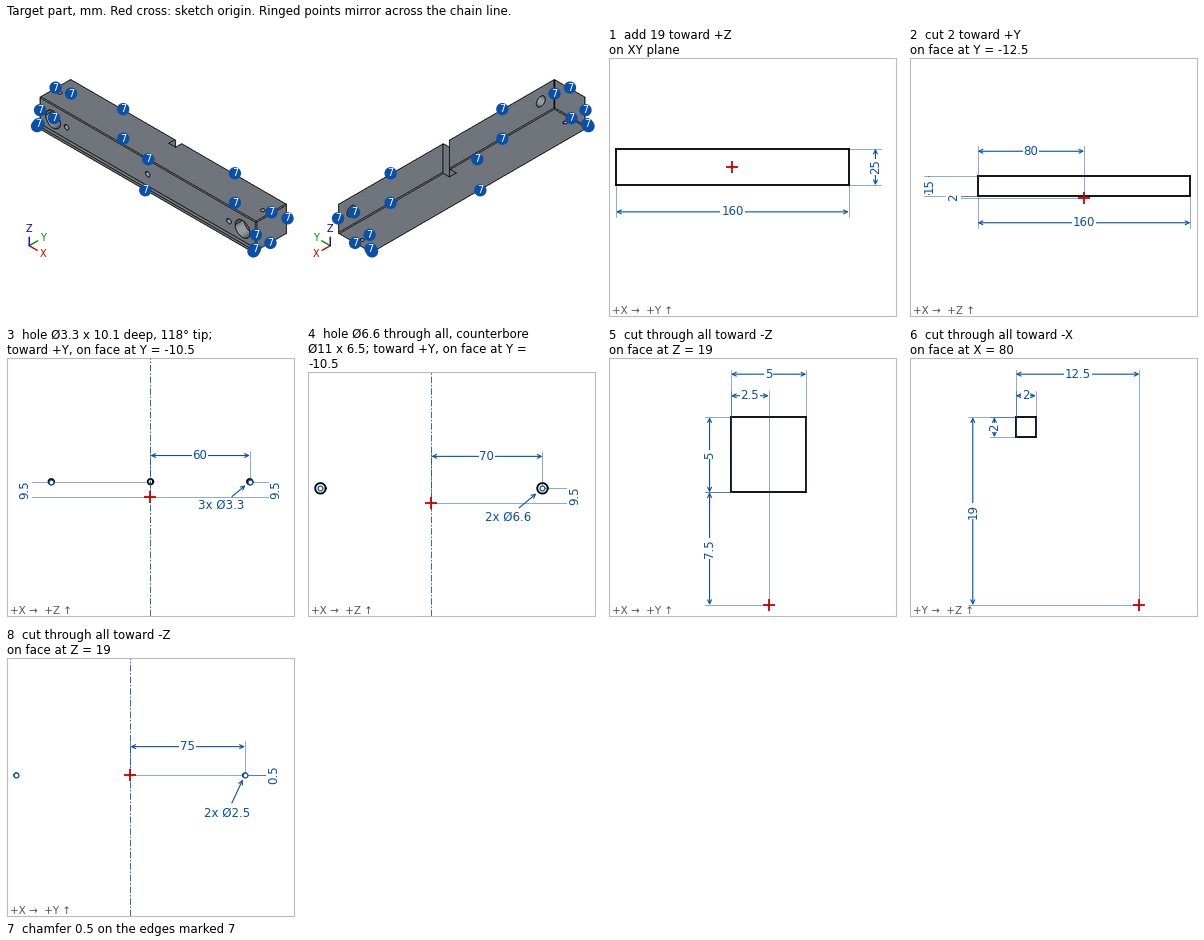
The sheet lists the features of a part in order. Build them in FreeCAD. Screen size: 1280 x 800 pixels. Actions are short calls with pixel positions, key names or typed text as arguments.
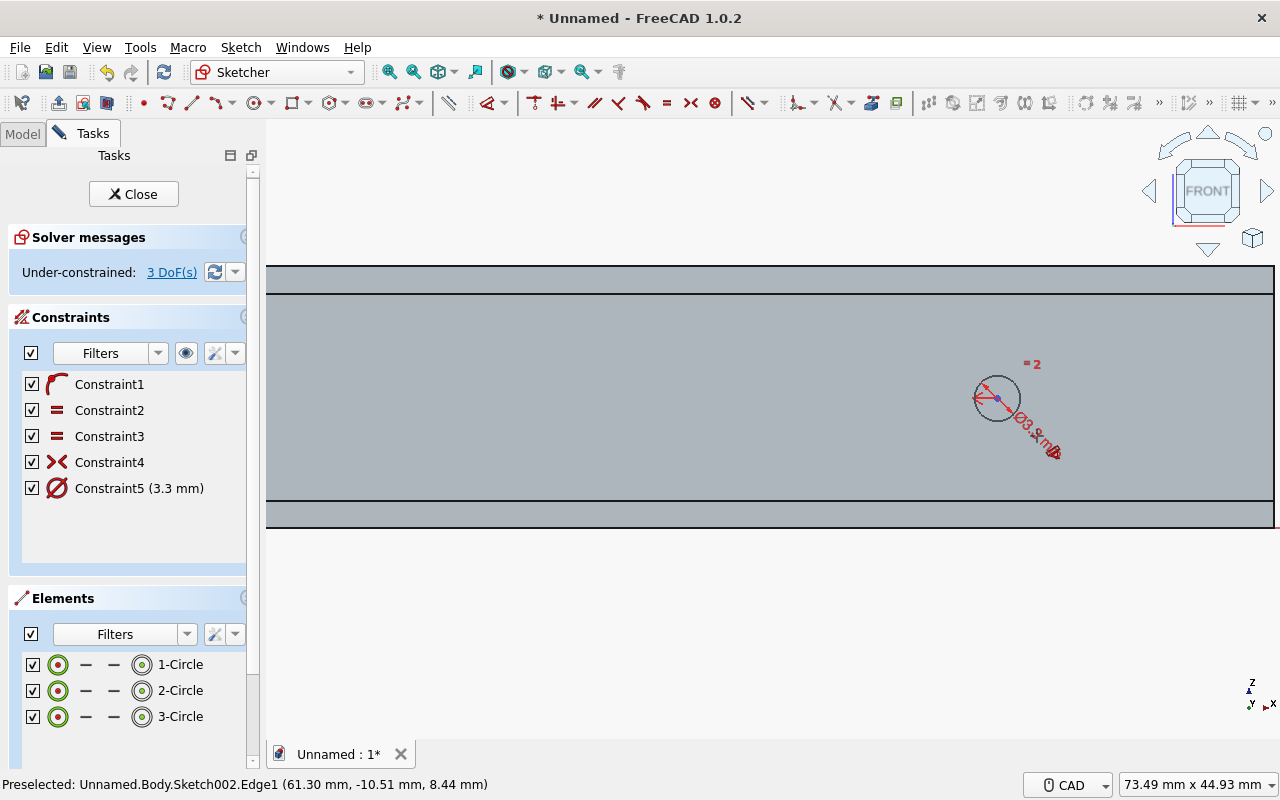
click(997, 398)
click(646, 562)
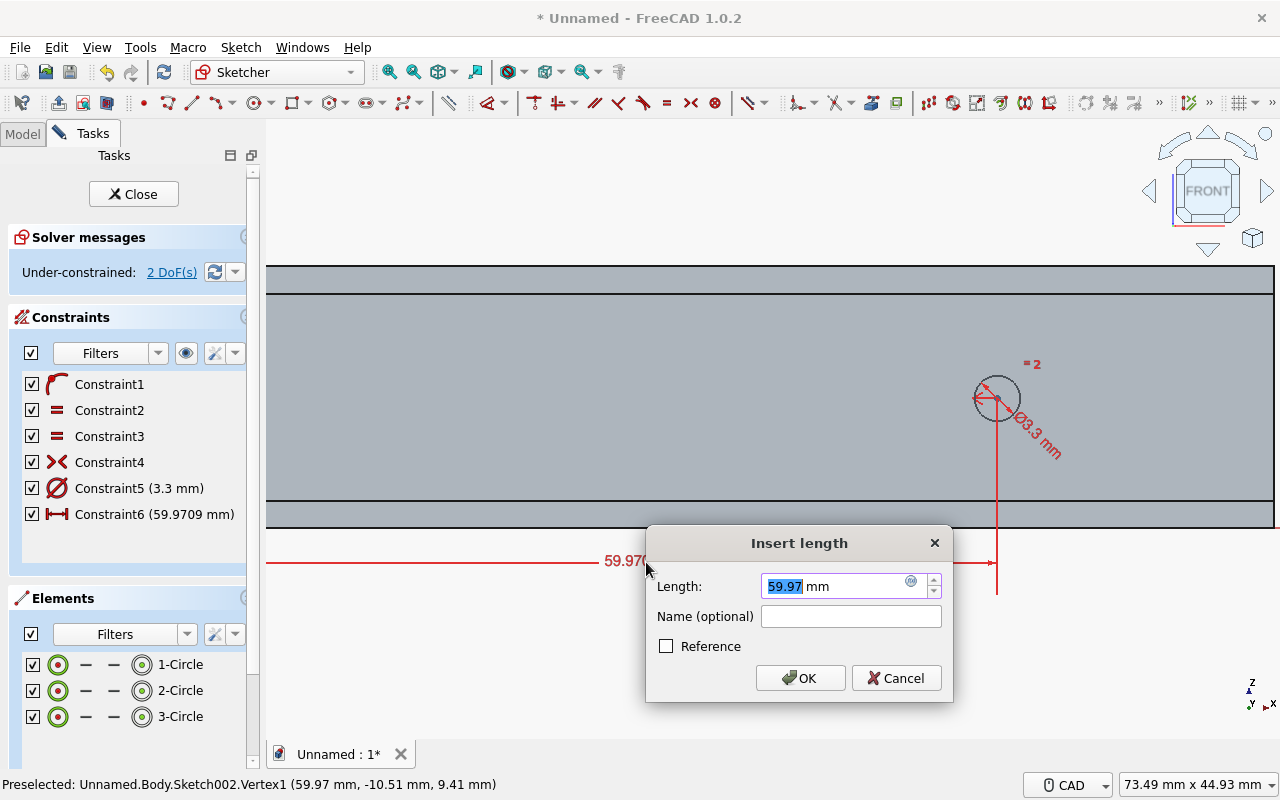
text(60)
key(Return)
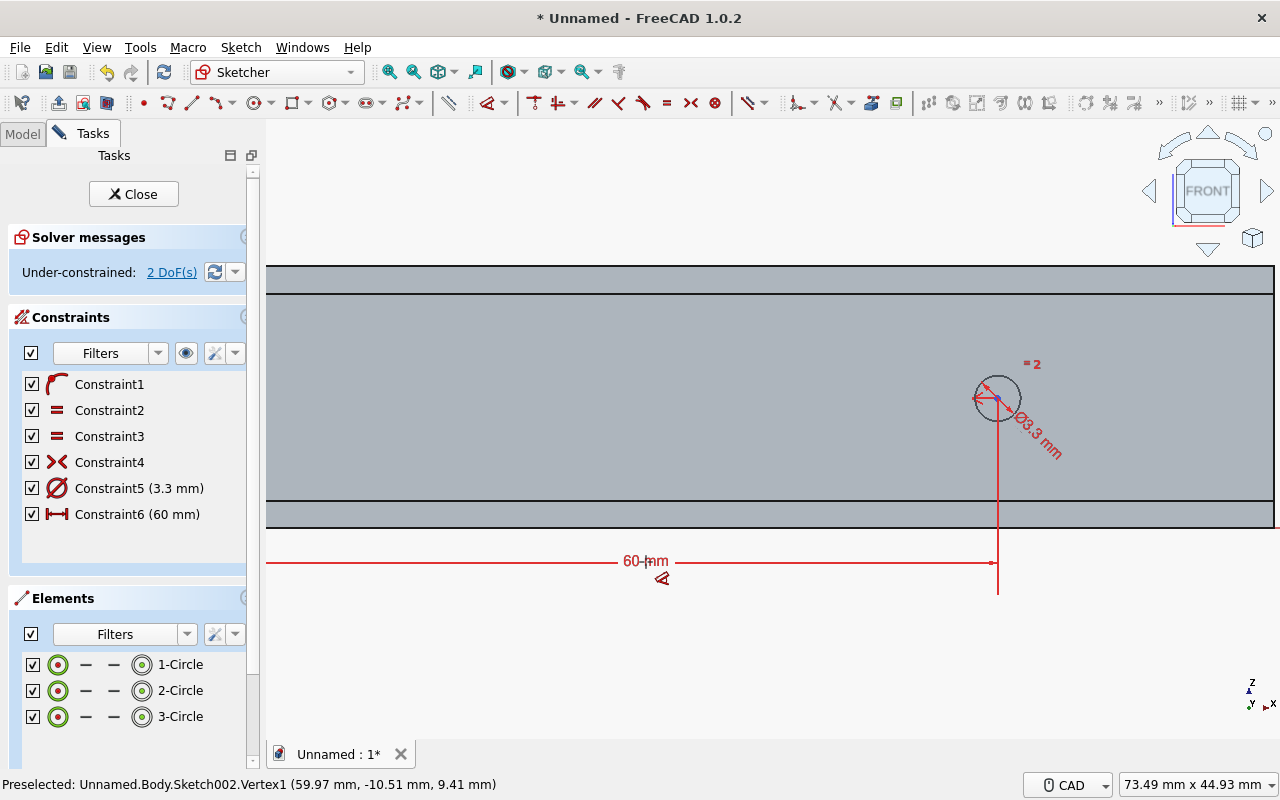
click(998, 398)
click(1032, 463)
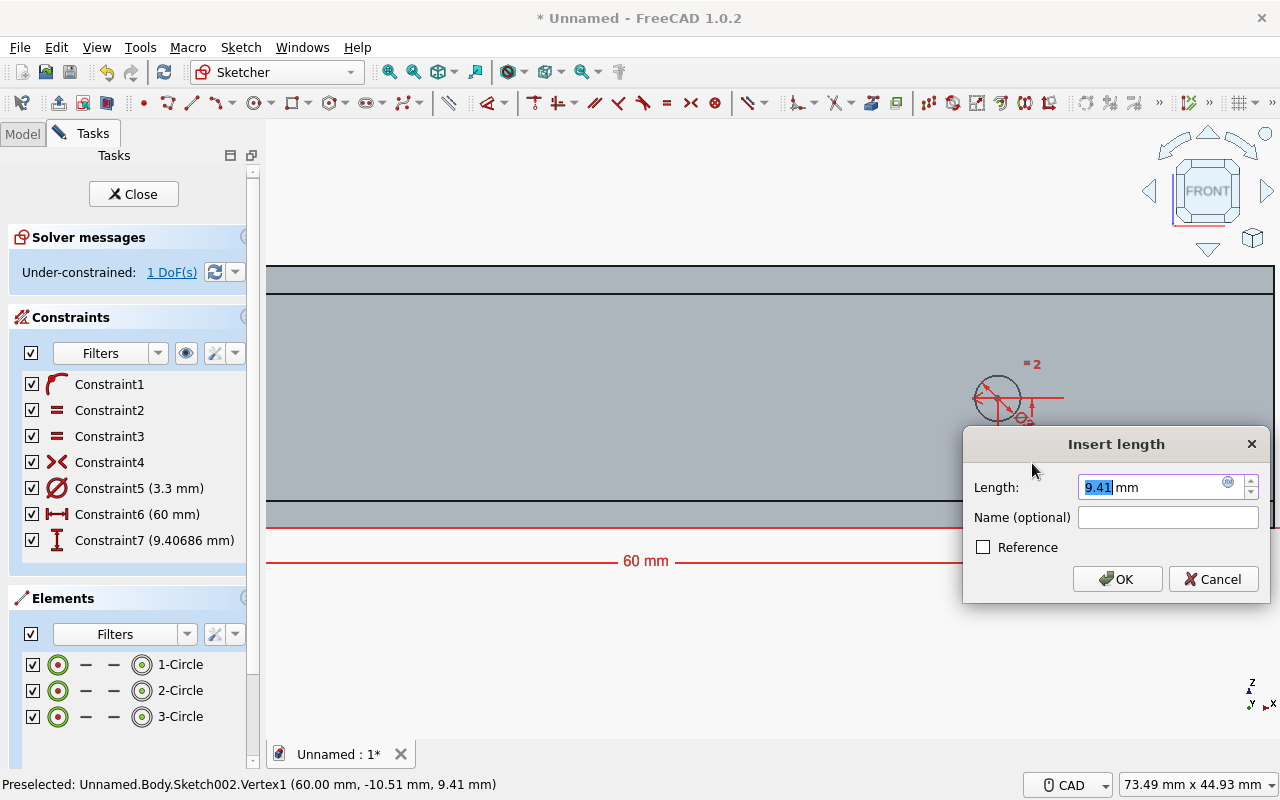
text(9.5)
key(Return)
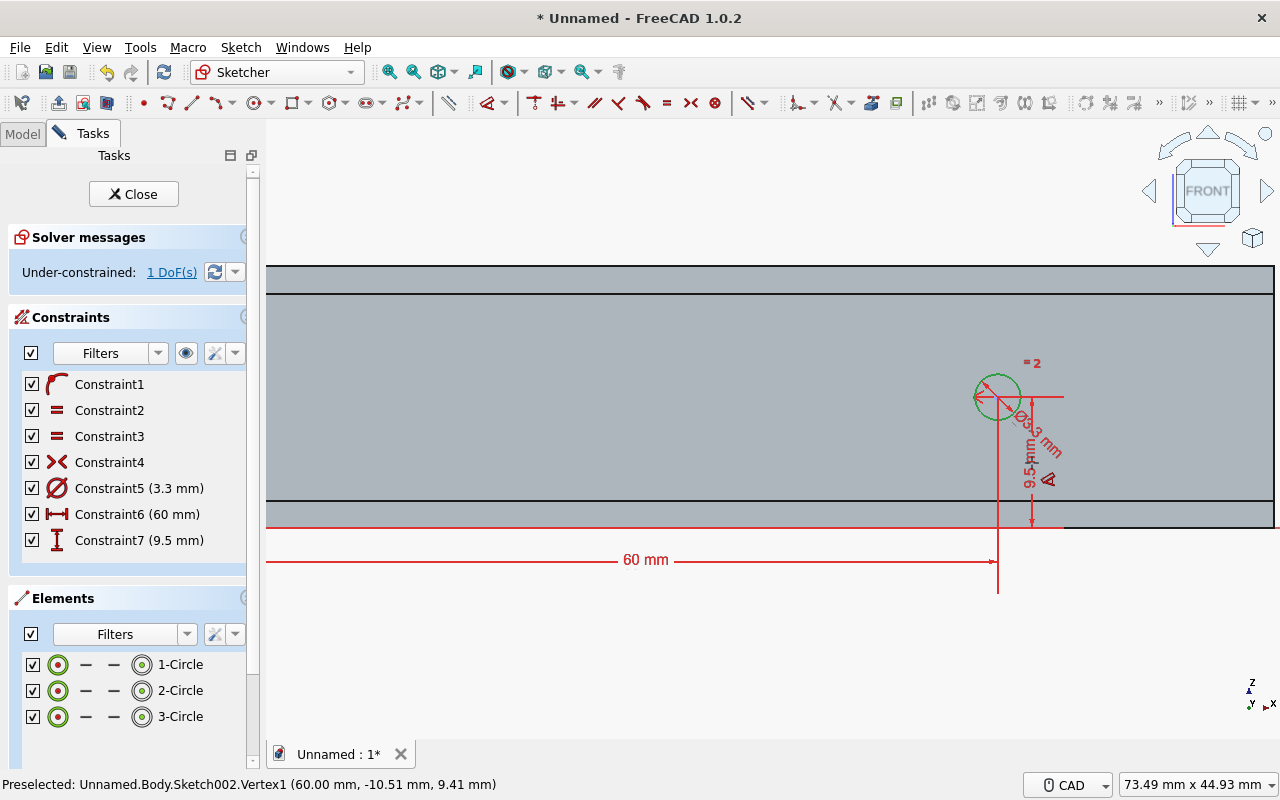
scroll(1016, 416, down, 5)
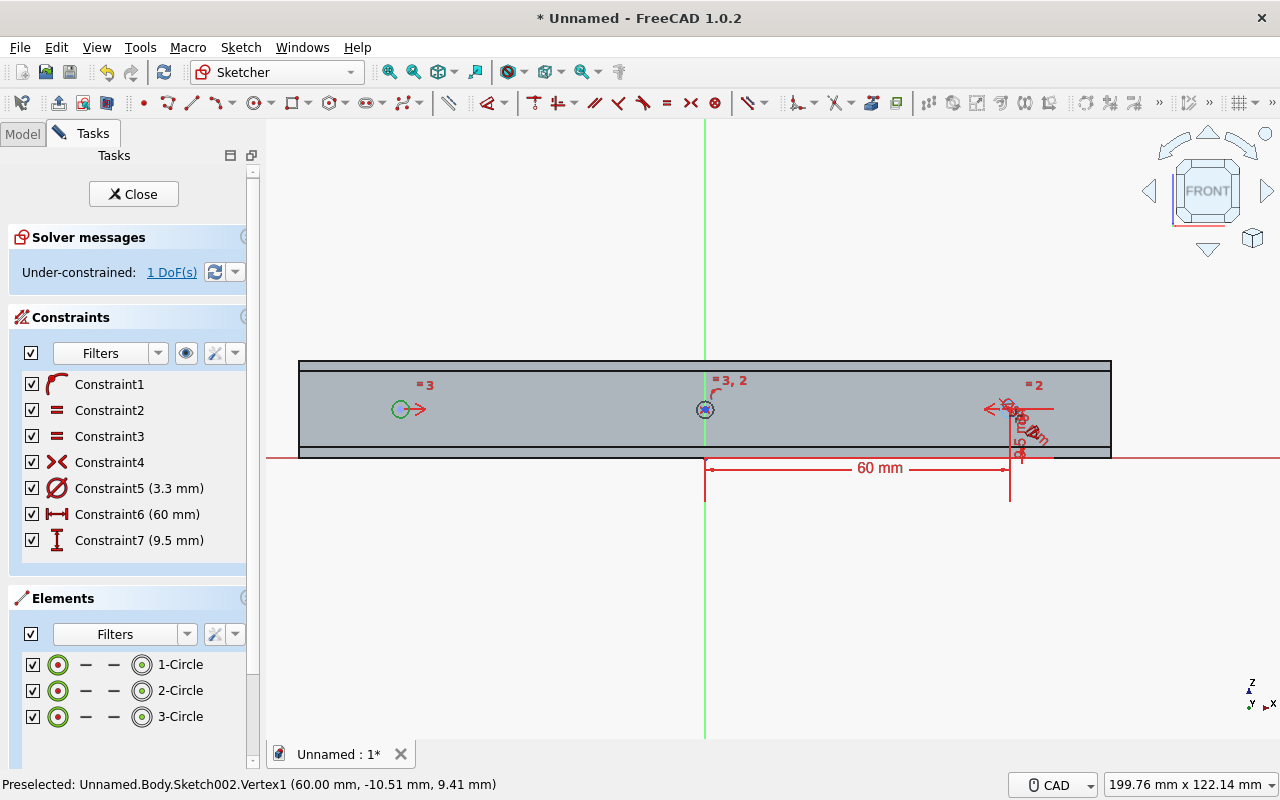
click(705, 410)
click(739, 434)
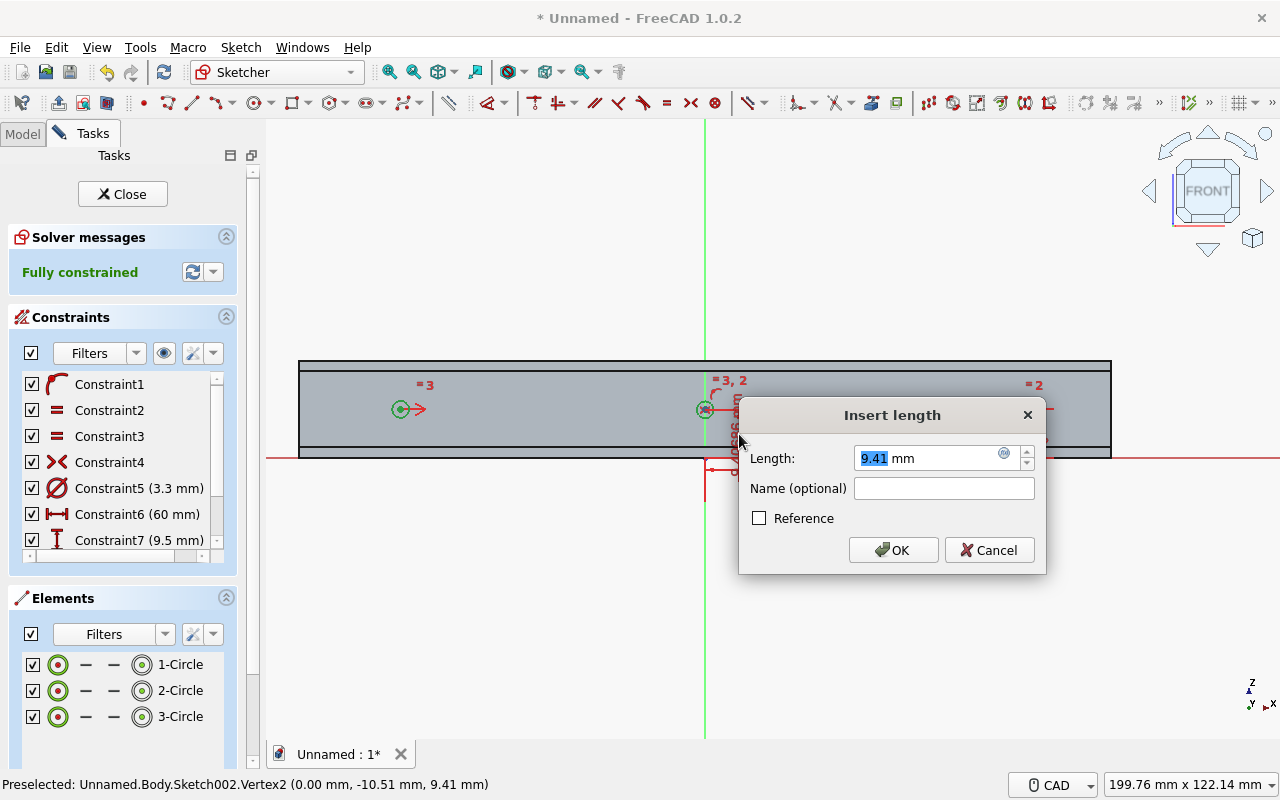
text(9.5)
key(Return)
key(Escape)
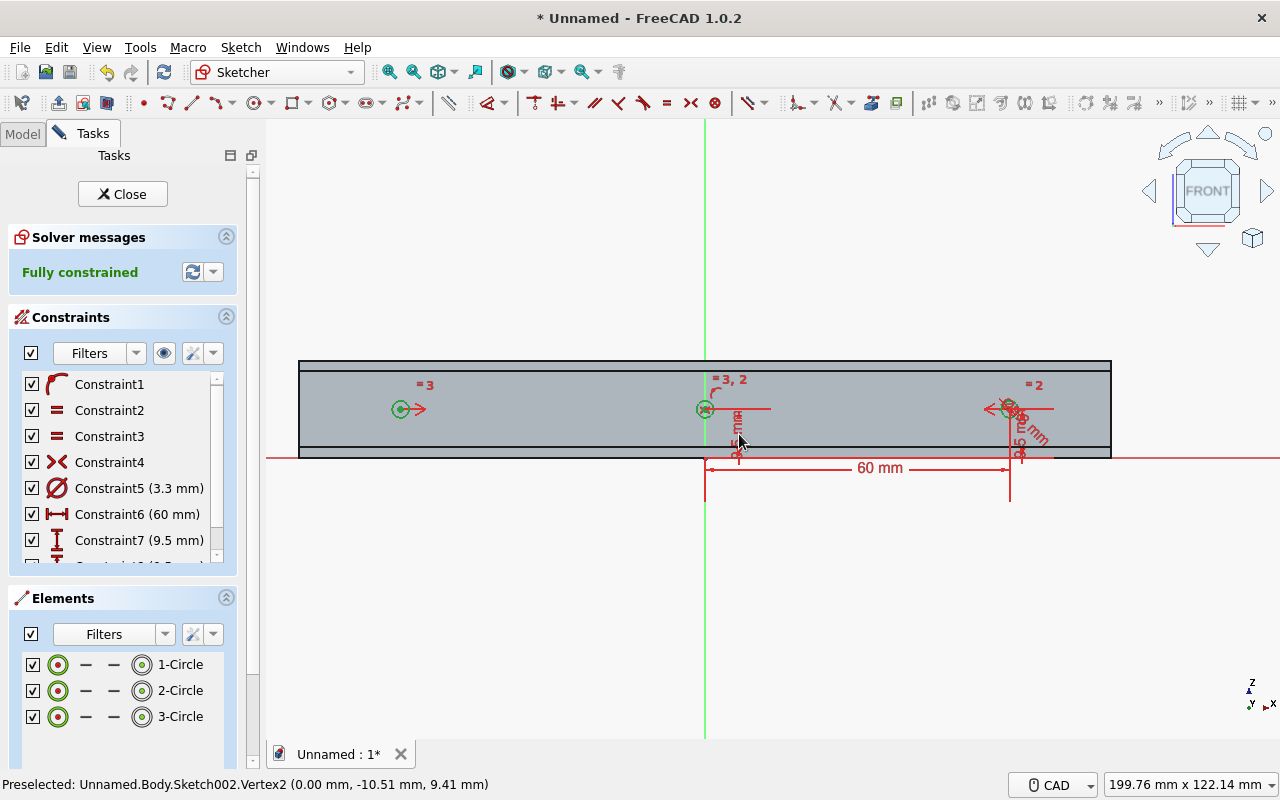
click(123, 194)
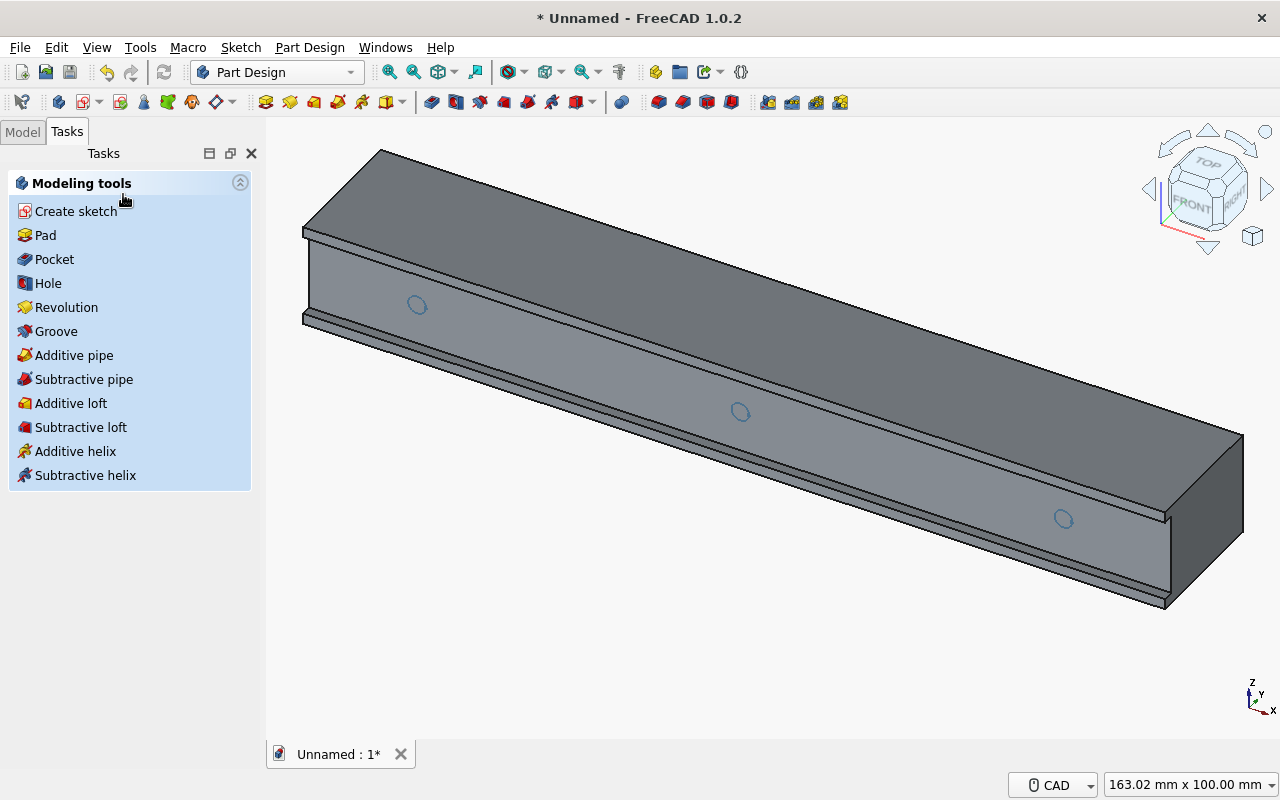
click(456, 102)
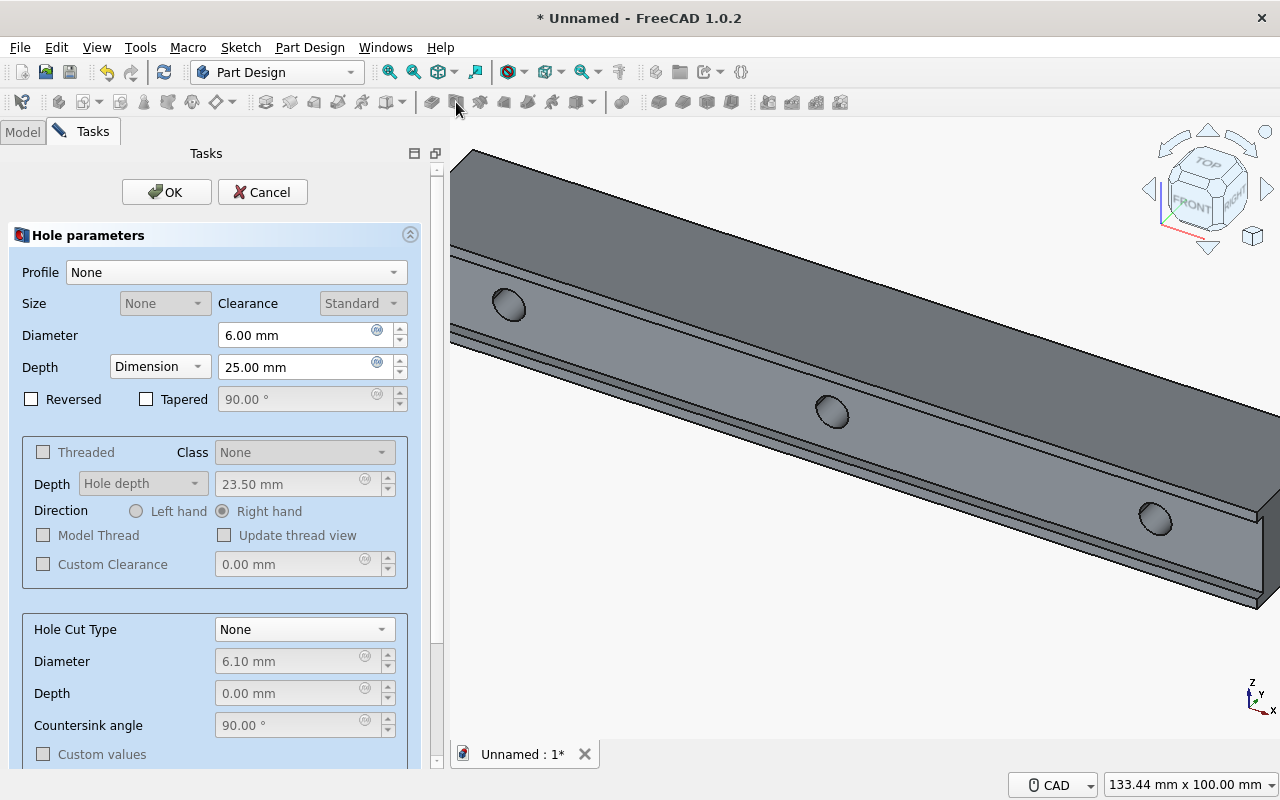
triple_click(305, 335)